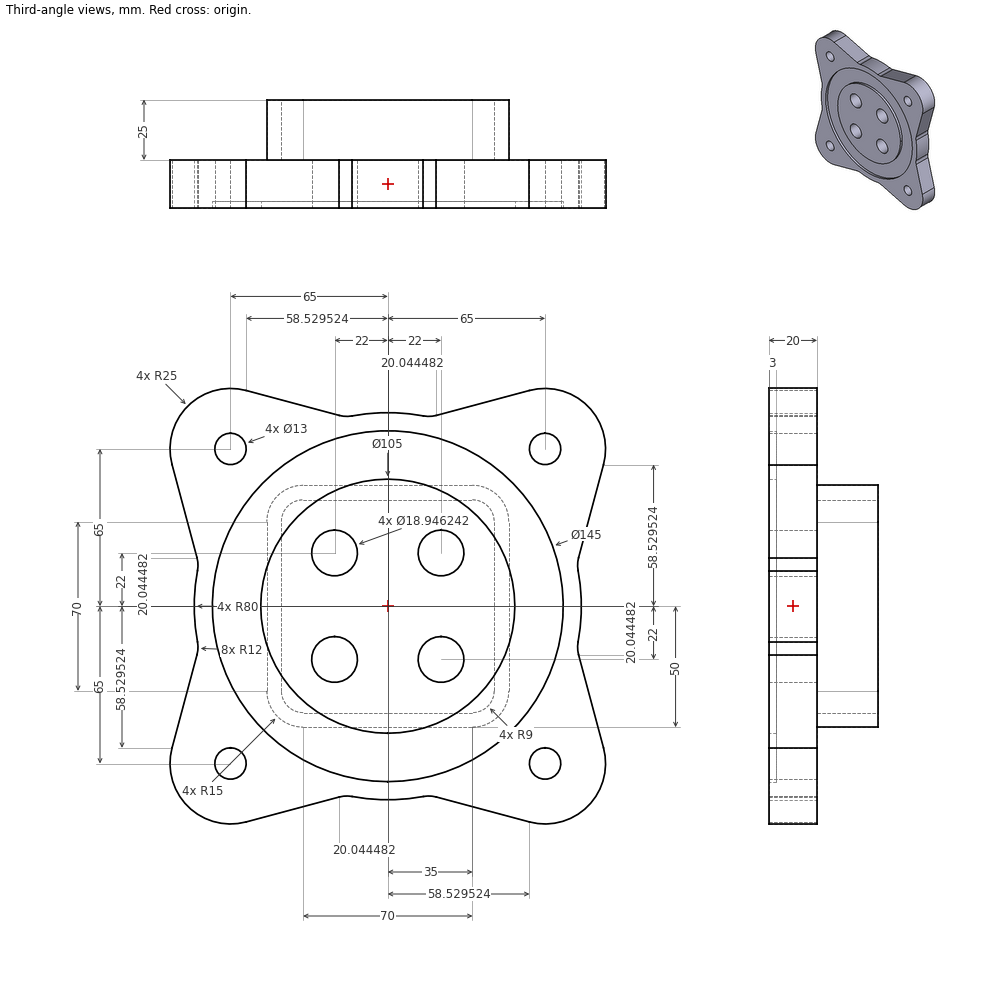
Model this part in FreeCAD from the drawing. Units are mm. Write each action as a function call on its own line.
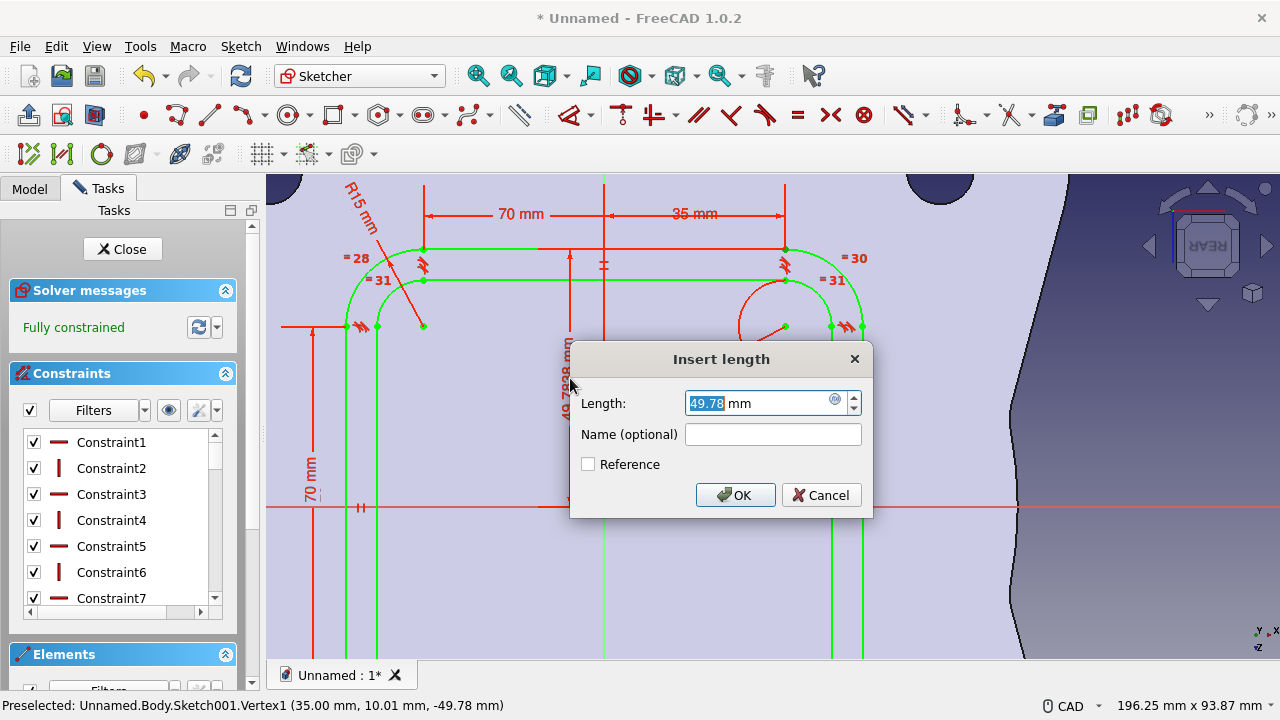
text(50)
key(Return)
key(Escape)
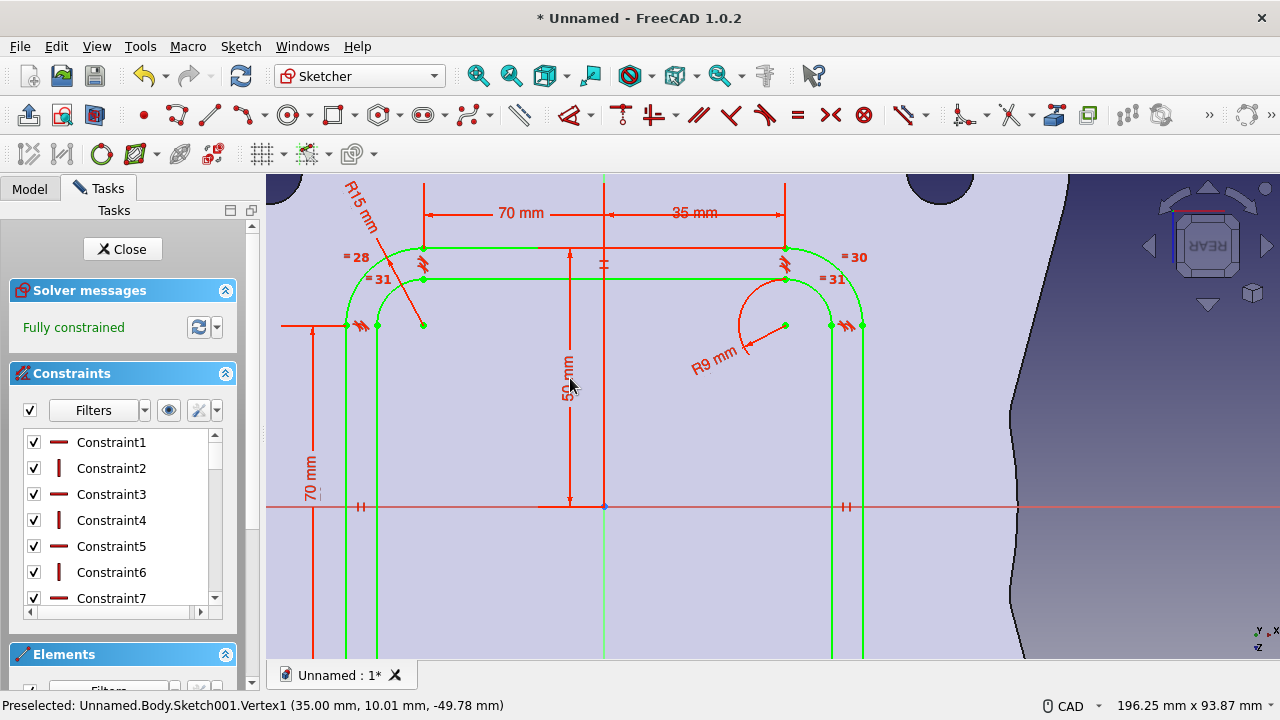
click(123, 249)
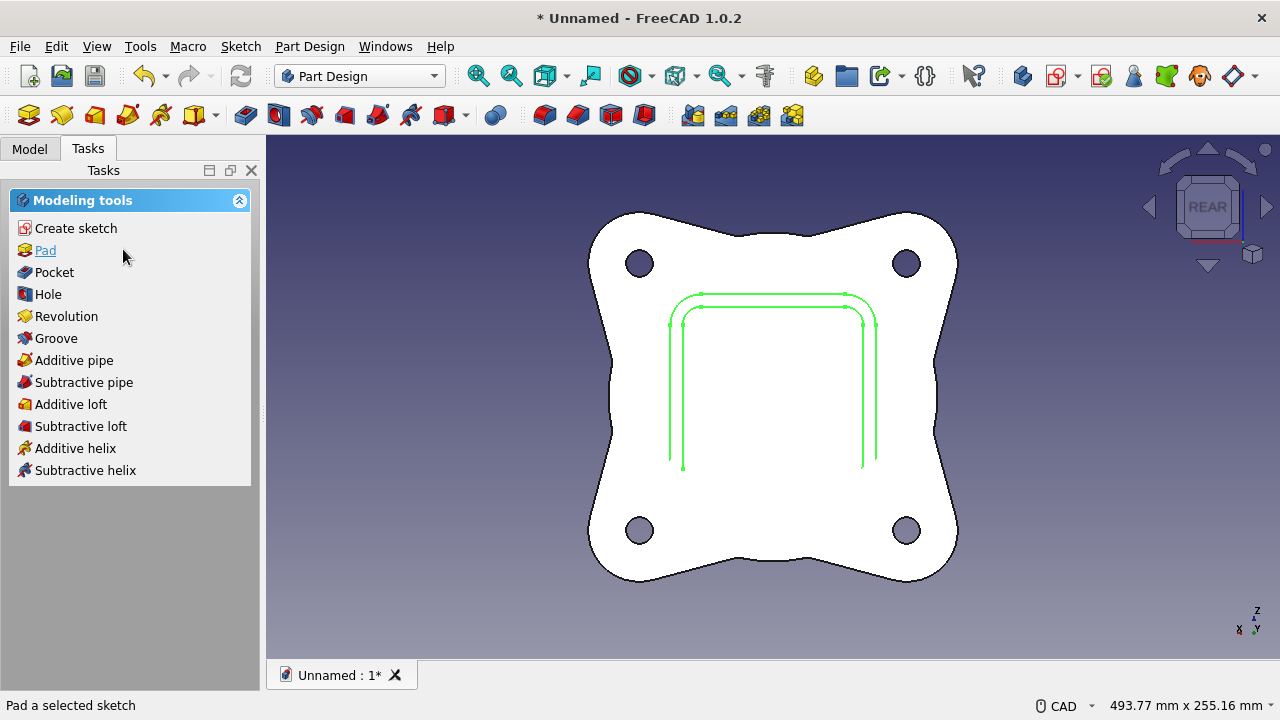
click(29, 116)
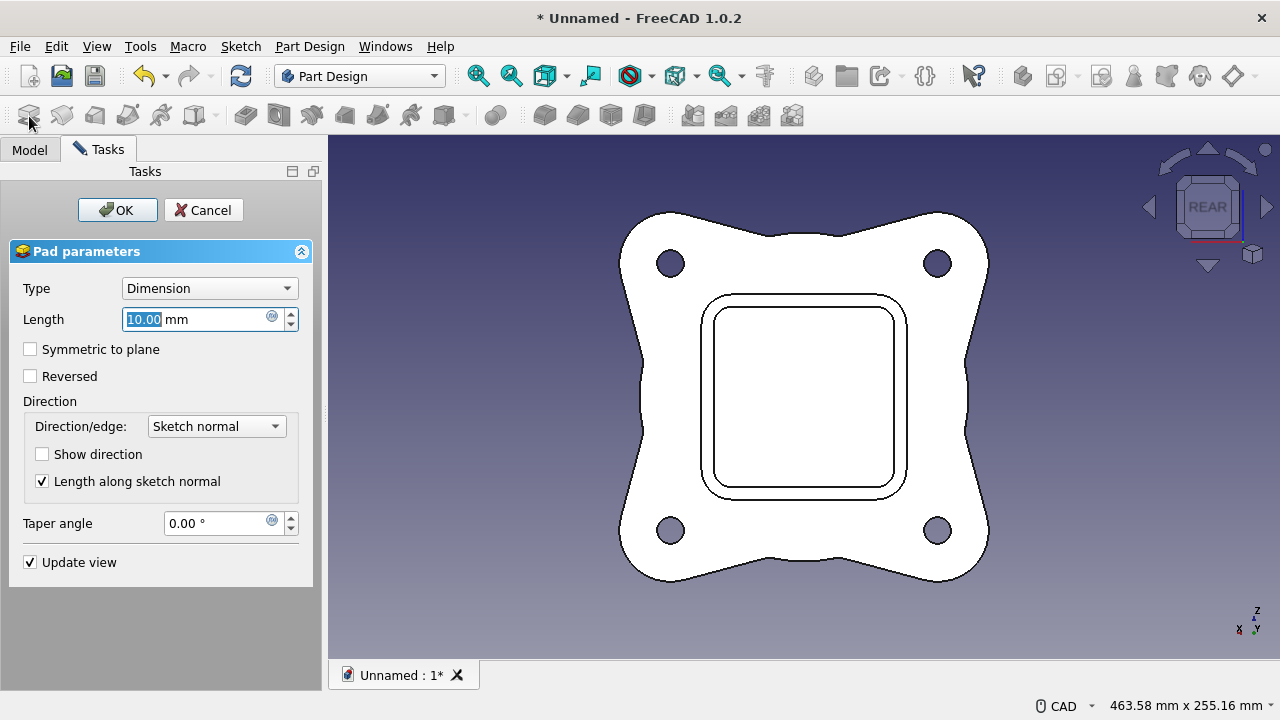
text(25)
key(Tab)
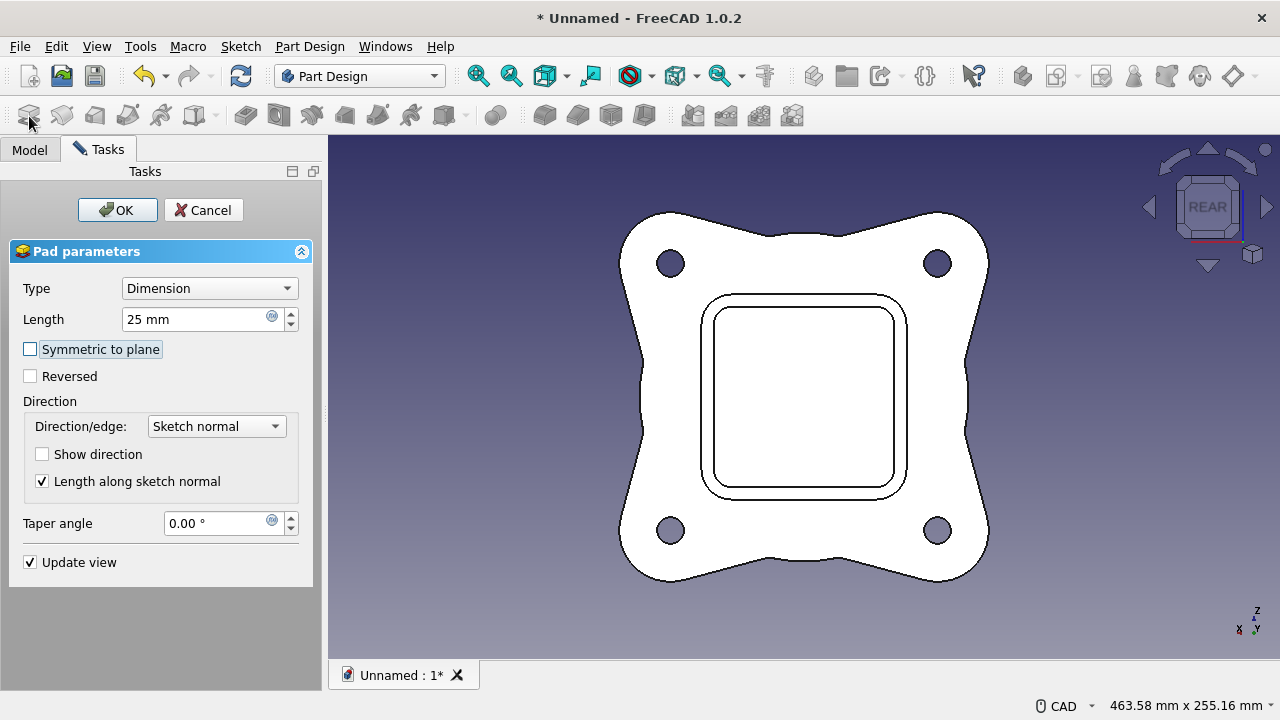
click(118, 210)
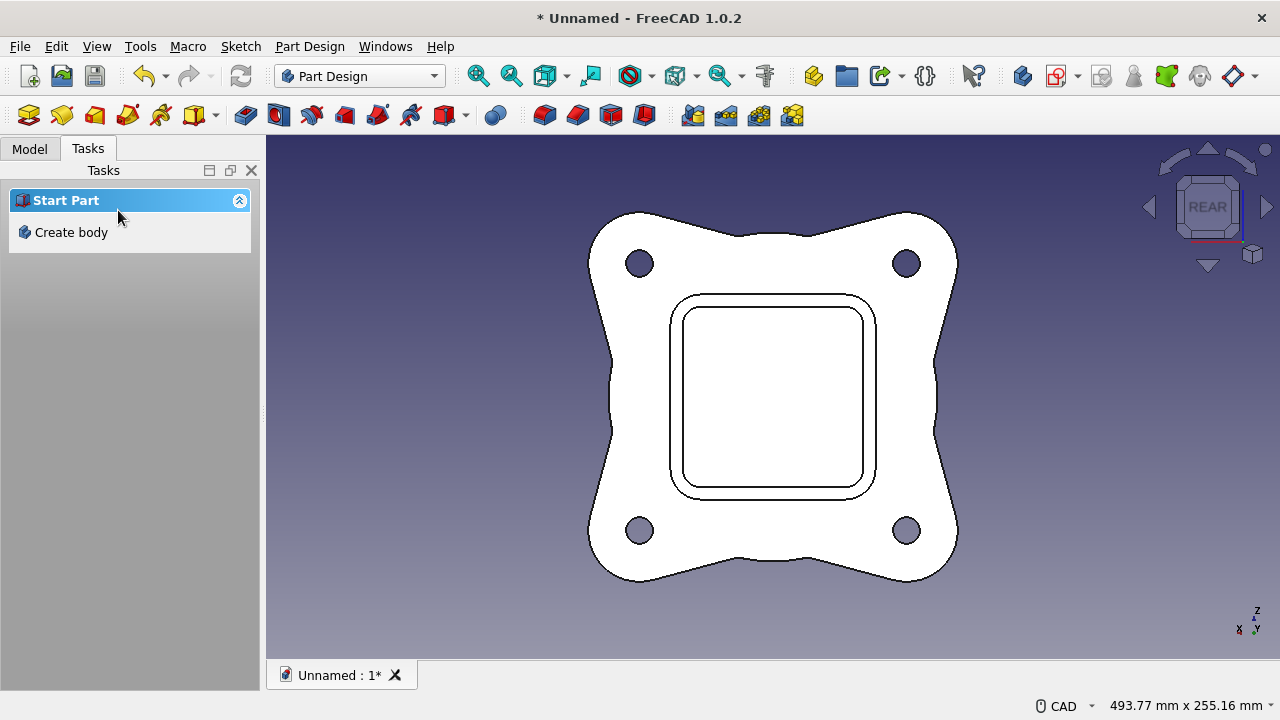
click(615, 290)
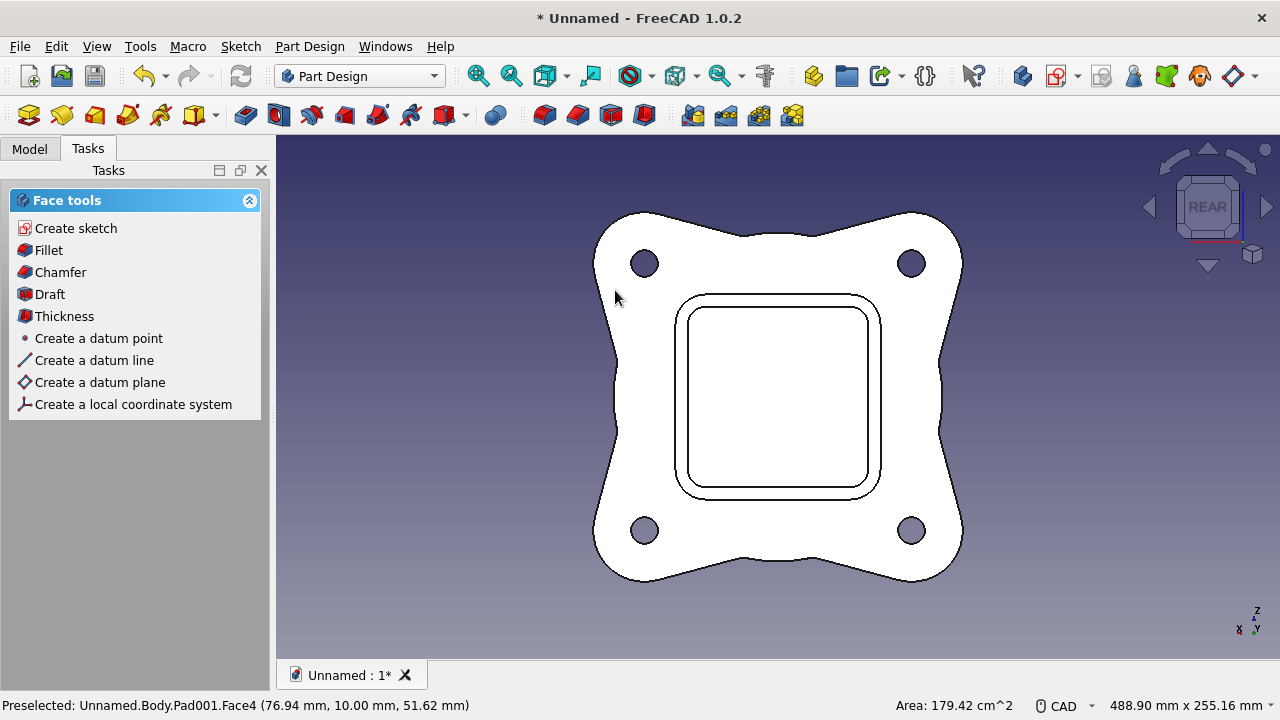
click(1056, 76)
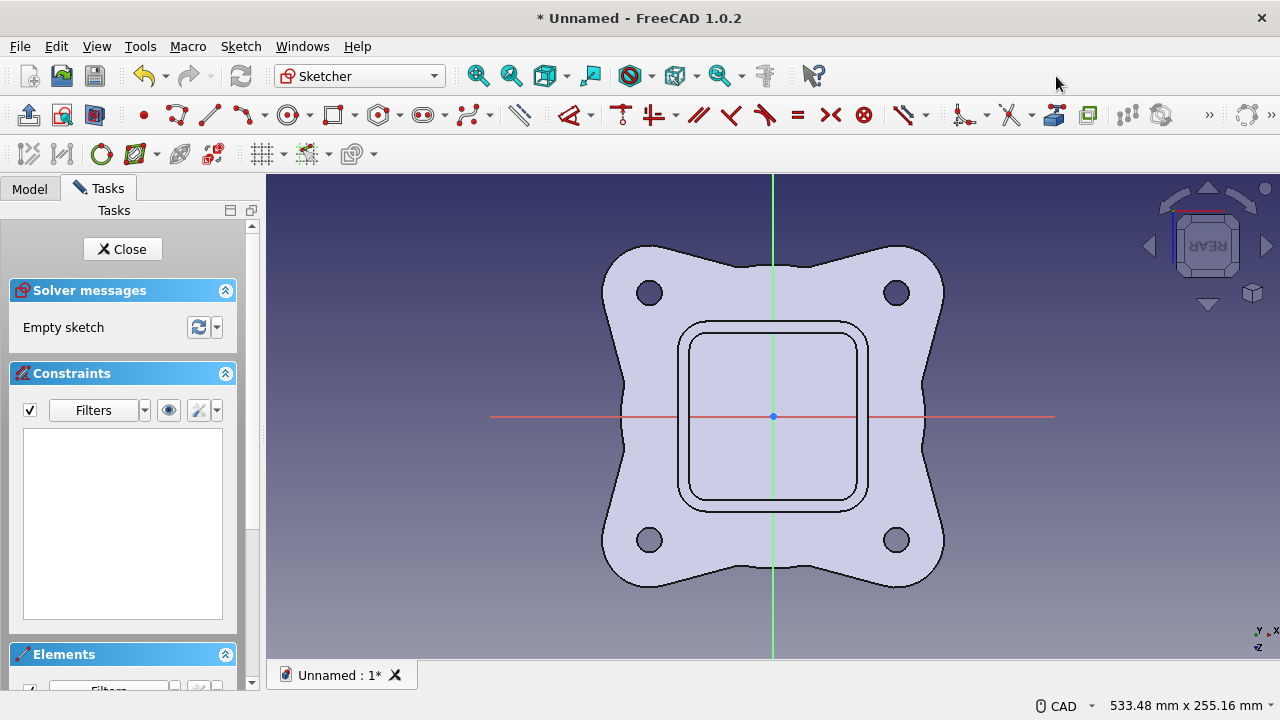
scroll(813, 416, up, 5)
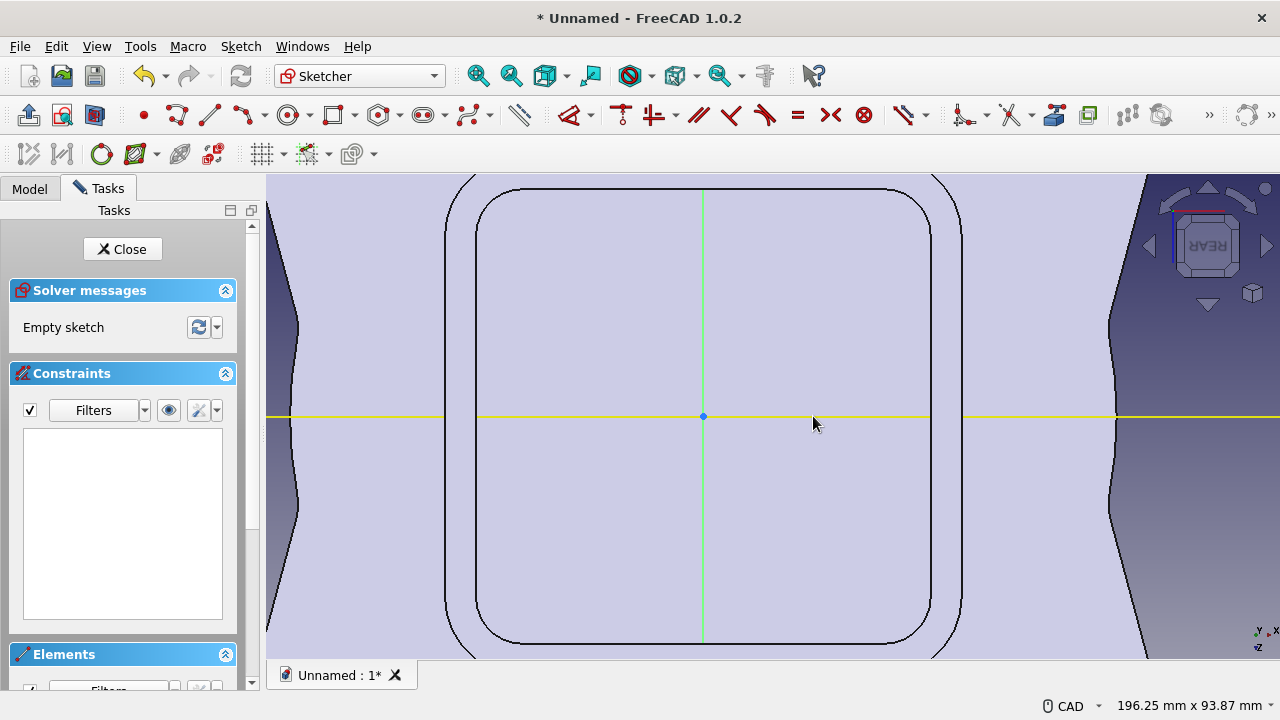
click(288, 116)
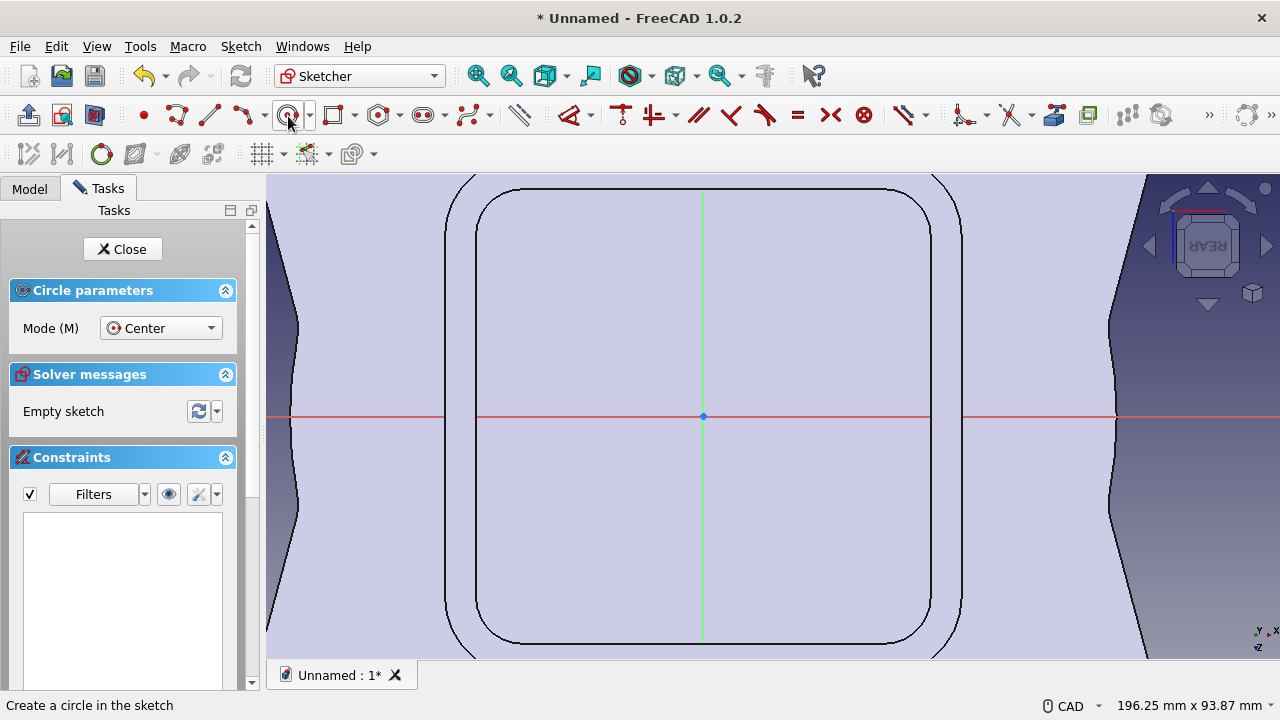
click(590, 530)
move(624, 496)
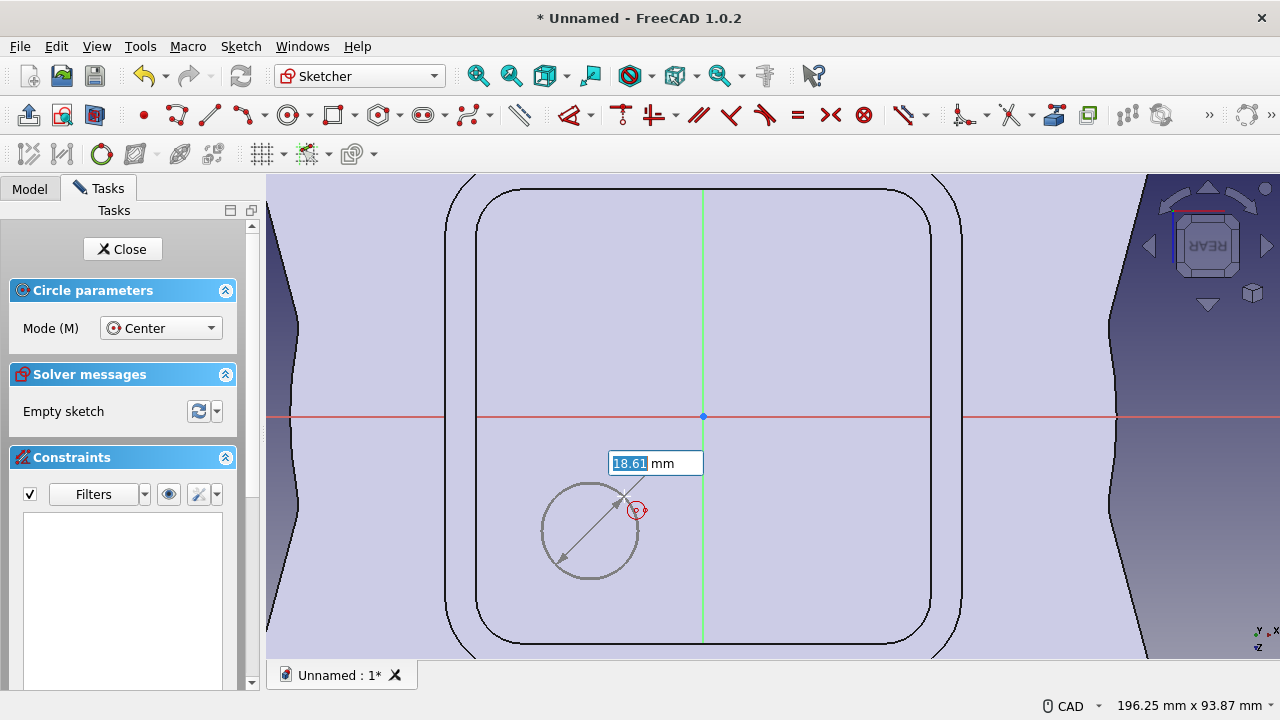
text(18.946242)
key(Return)